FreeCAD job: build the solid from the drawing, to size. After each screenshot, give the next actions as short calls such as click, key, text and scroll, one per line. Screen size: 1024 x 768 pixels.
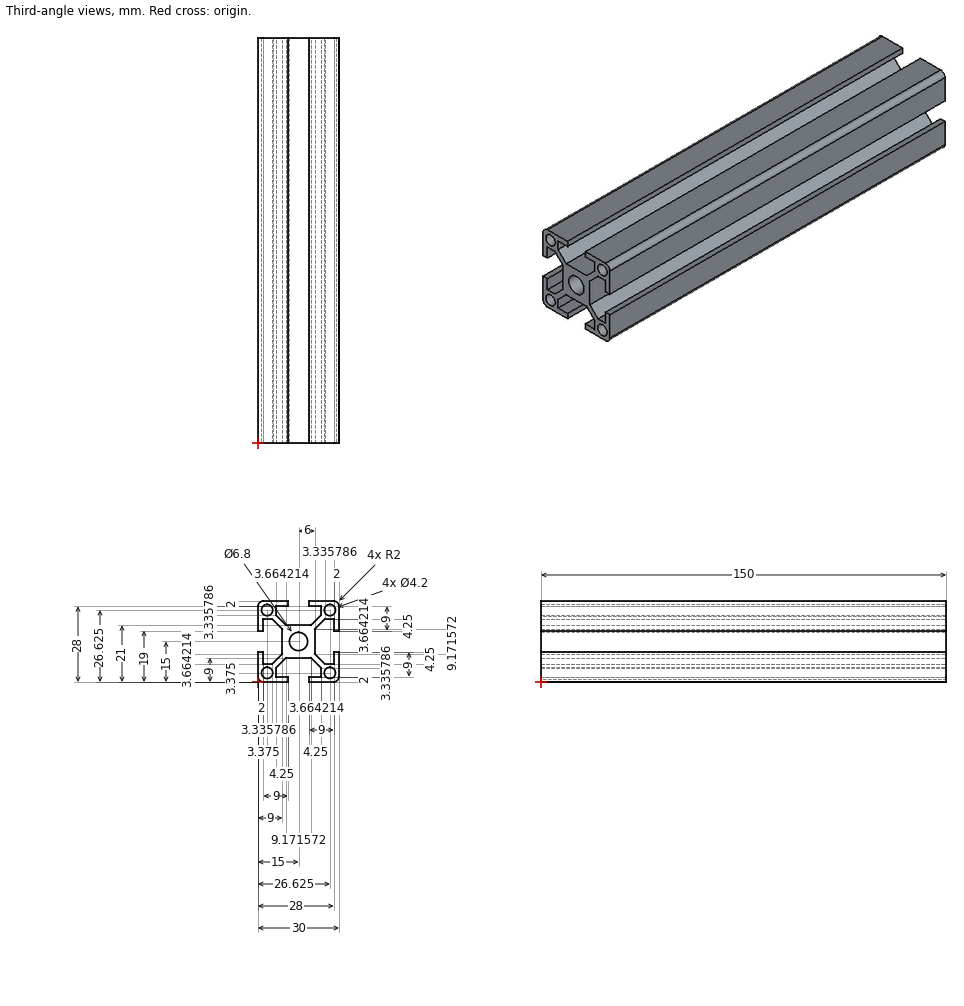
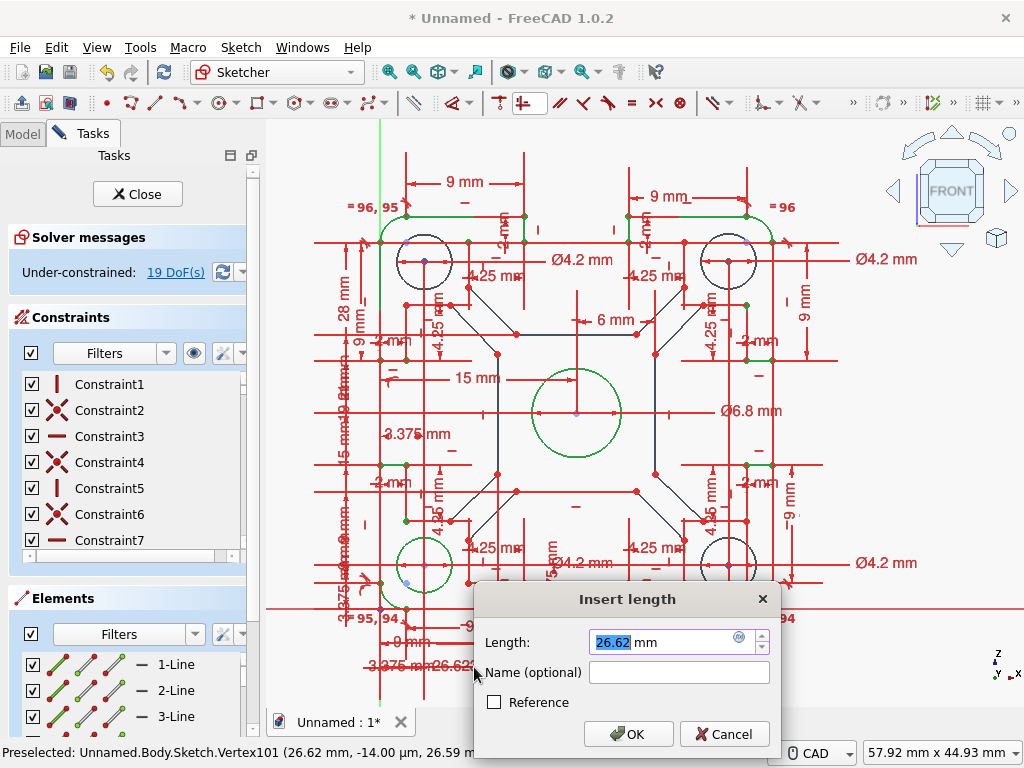
text(26.625)
key(Return)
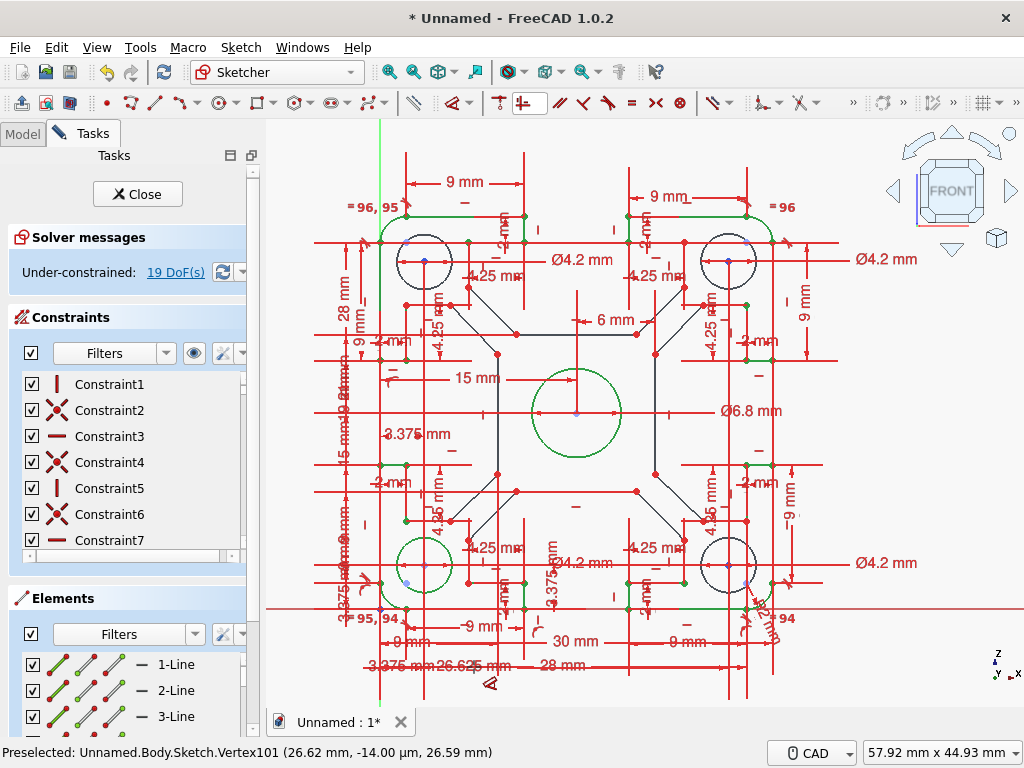
click(729, 261)
click(763, 435)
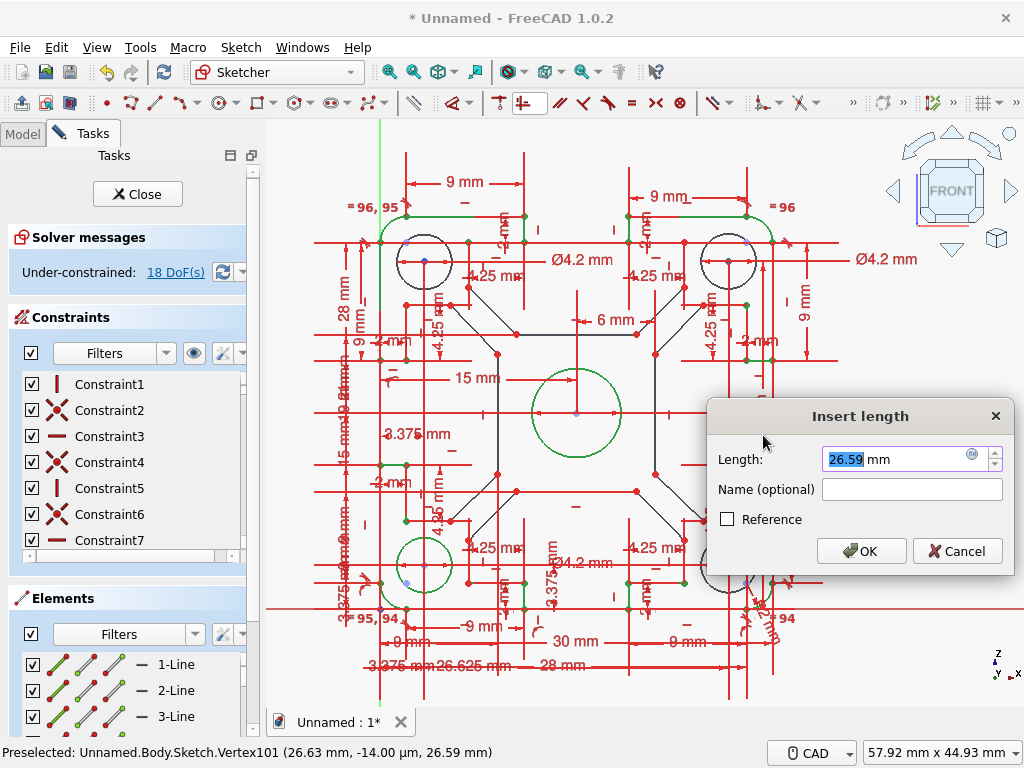
text(26.625)
key(Return)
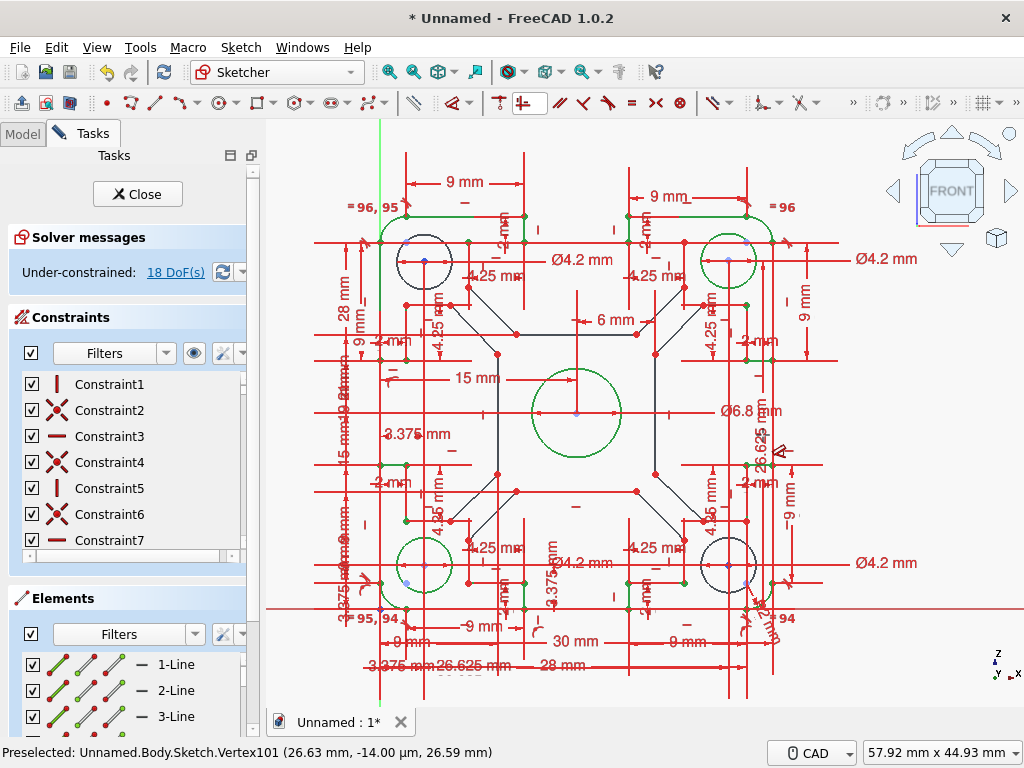
click(424, 262)
click(322, 356)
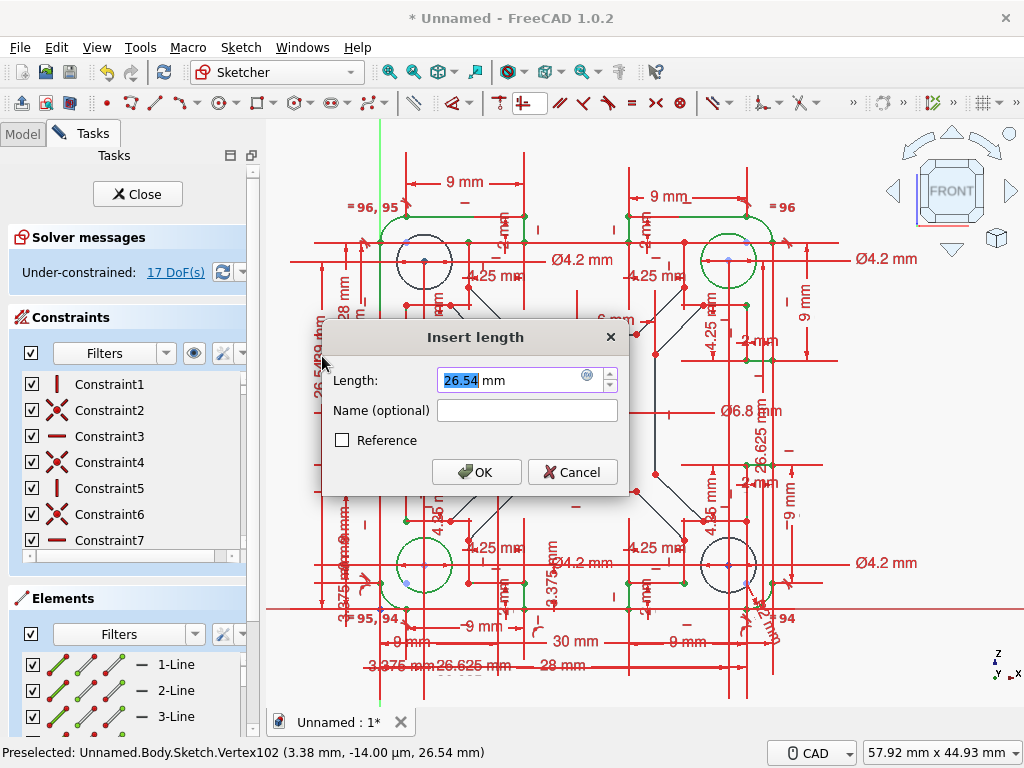
text(26.625)
key(Return)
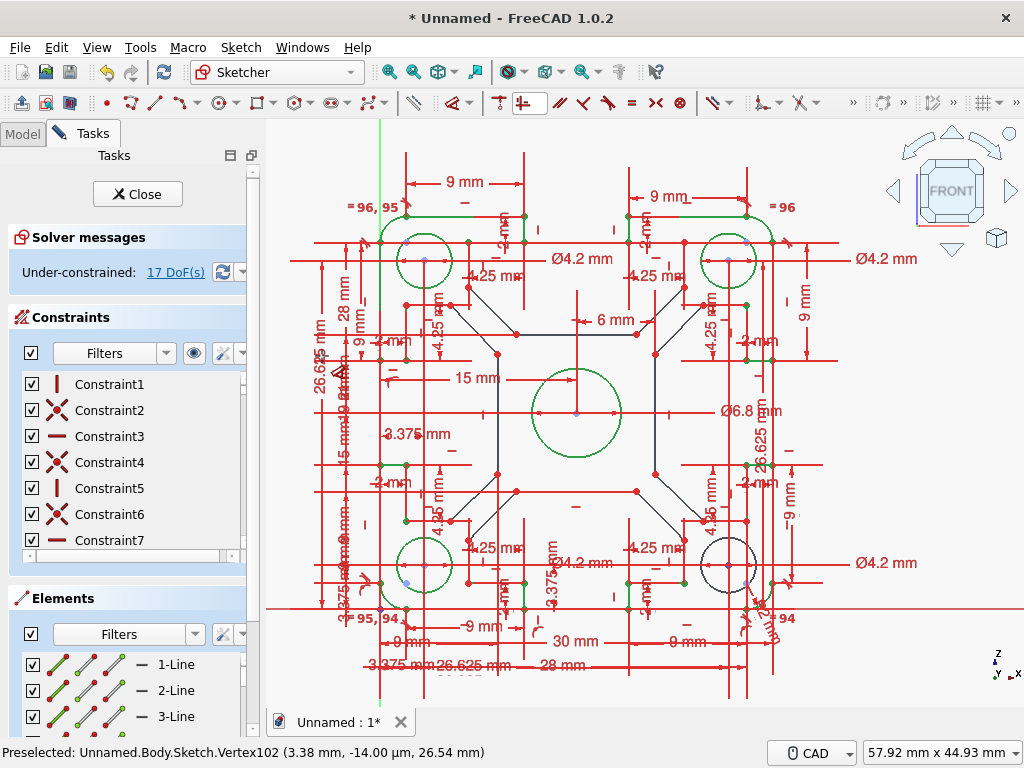
click(729, 565)
click(634, 667)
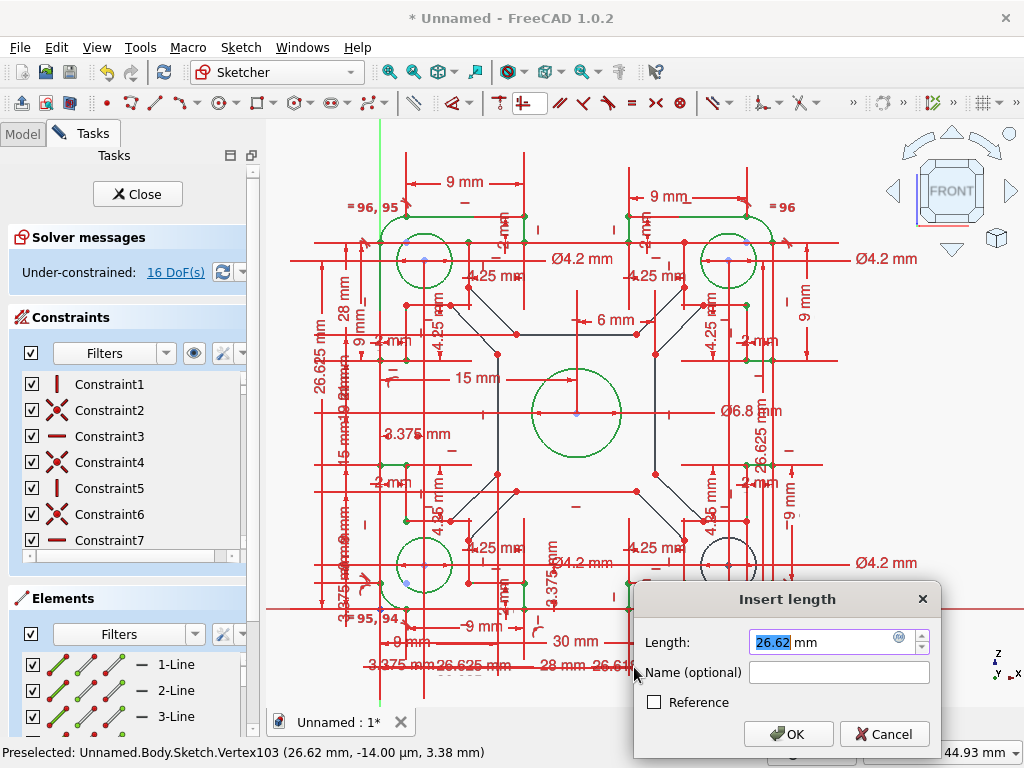
text(26.625)
key(Return)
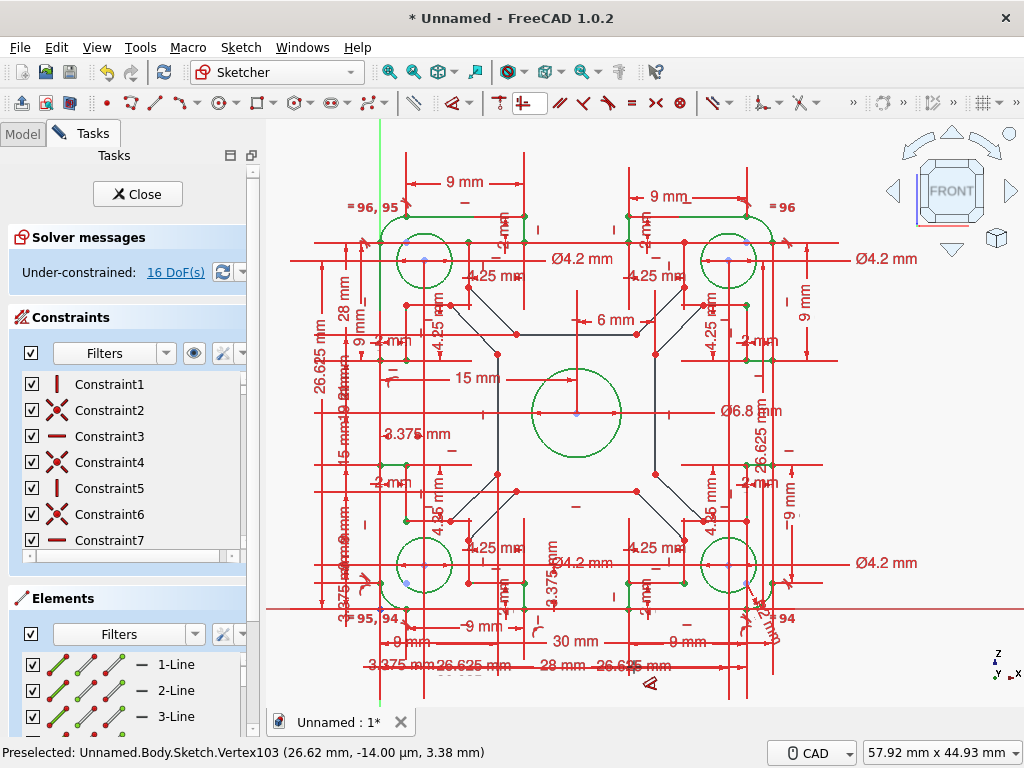
click(734, 305)
click(735, 271)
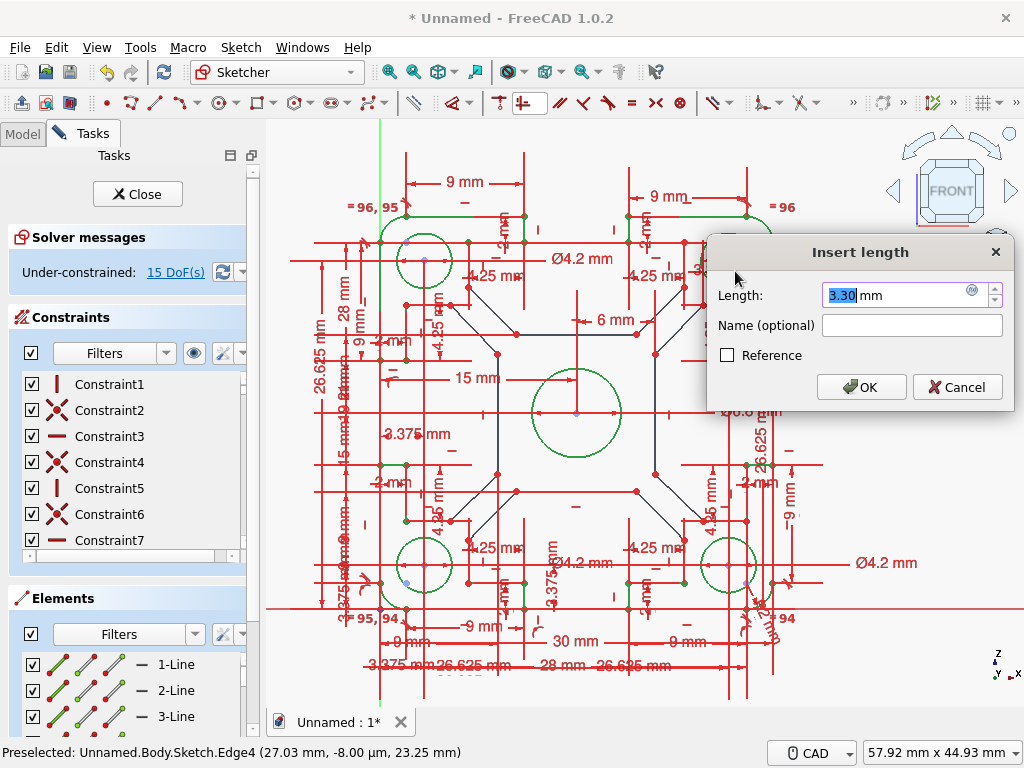
text(3.335786)
key(Return)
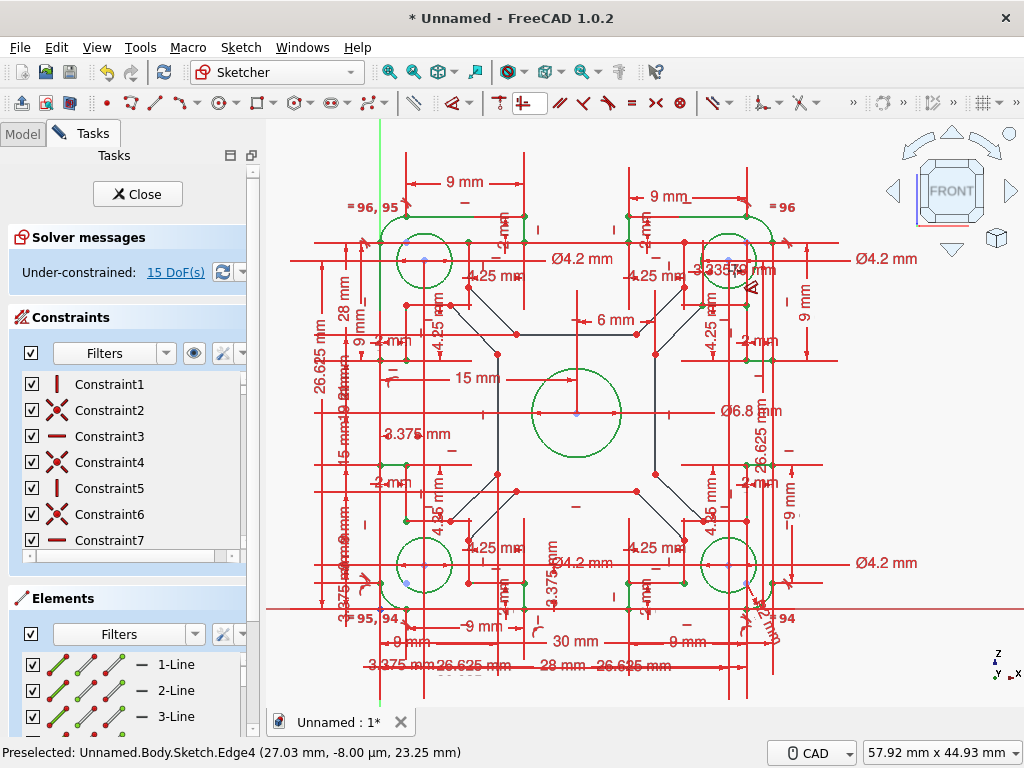
click(655, 391)
click(689, 415)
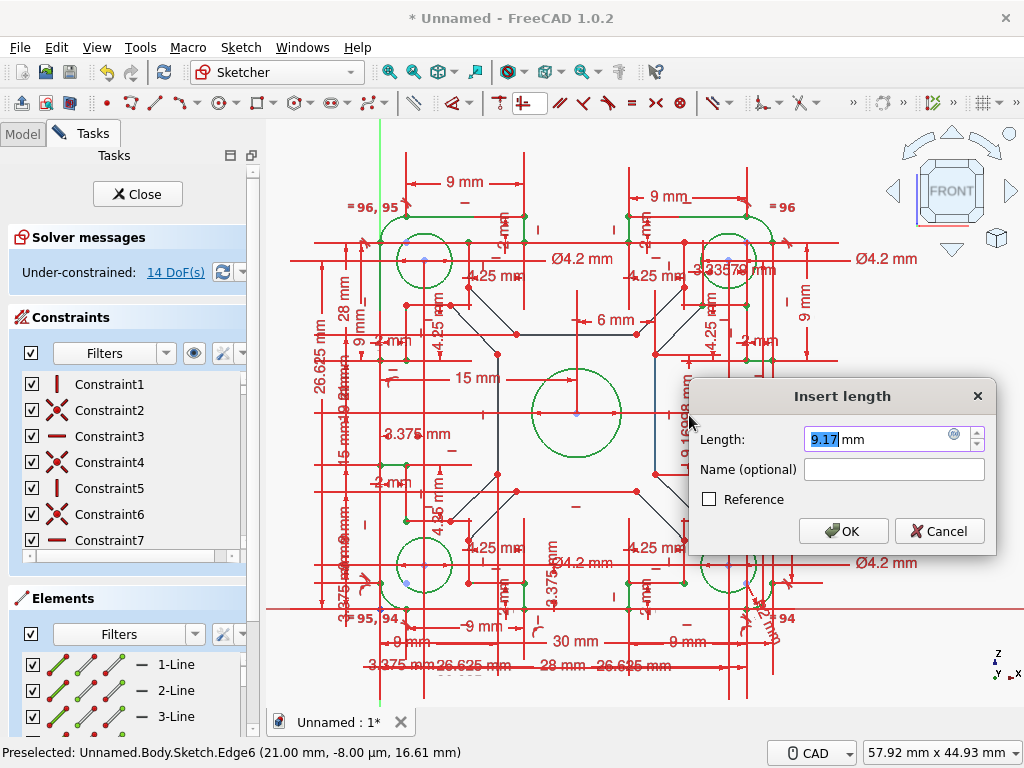
text(9.171572)
key(Return)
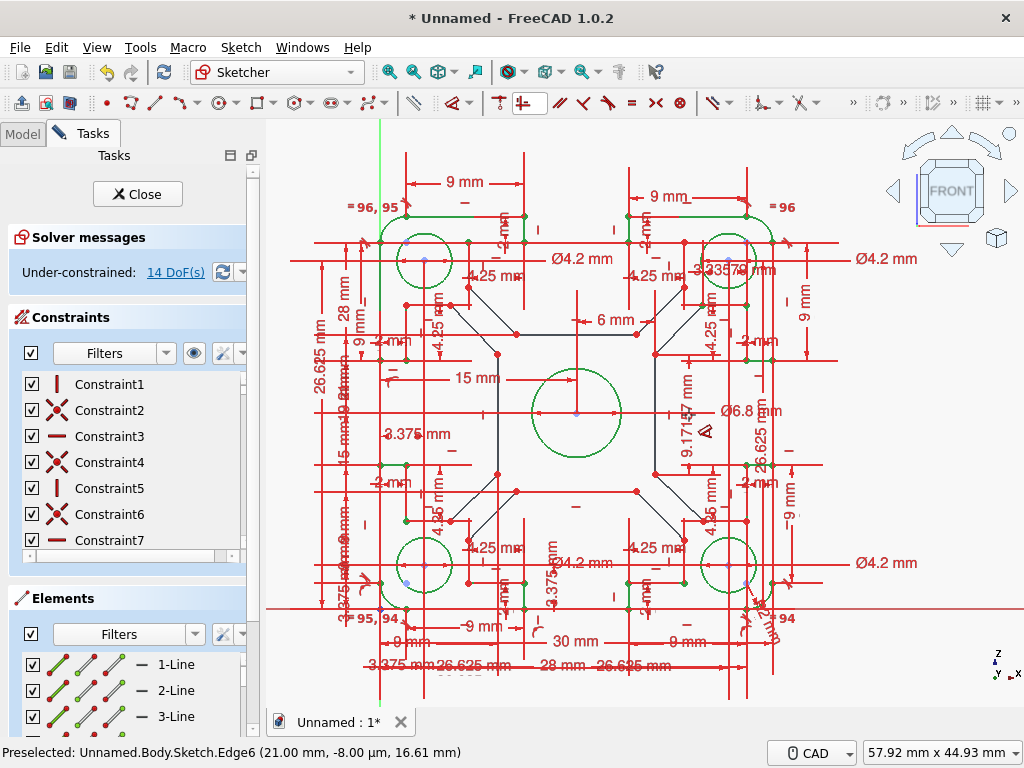
click(716, 521)
click(735, 555)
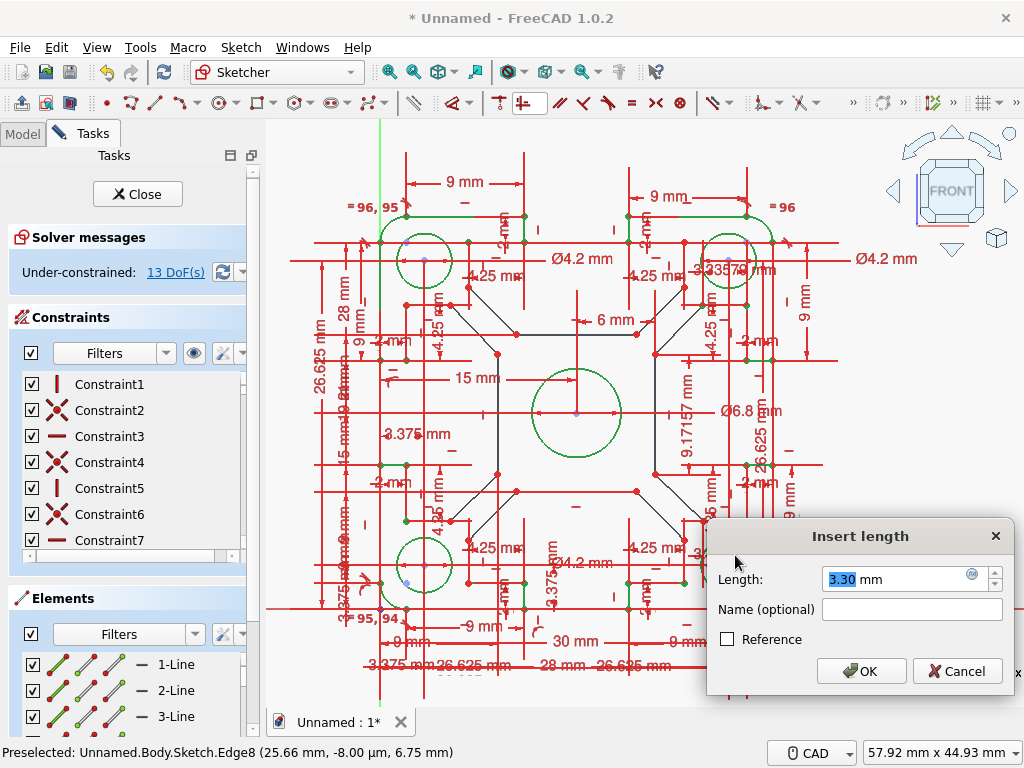
text(3.335786)
key(Return)